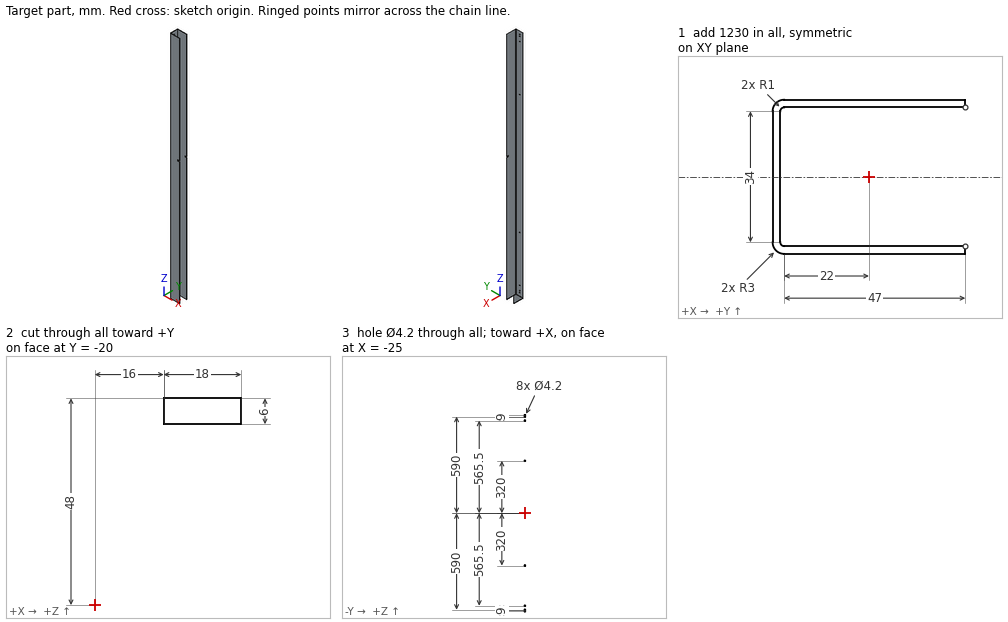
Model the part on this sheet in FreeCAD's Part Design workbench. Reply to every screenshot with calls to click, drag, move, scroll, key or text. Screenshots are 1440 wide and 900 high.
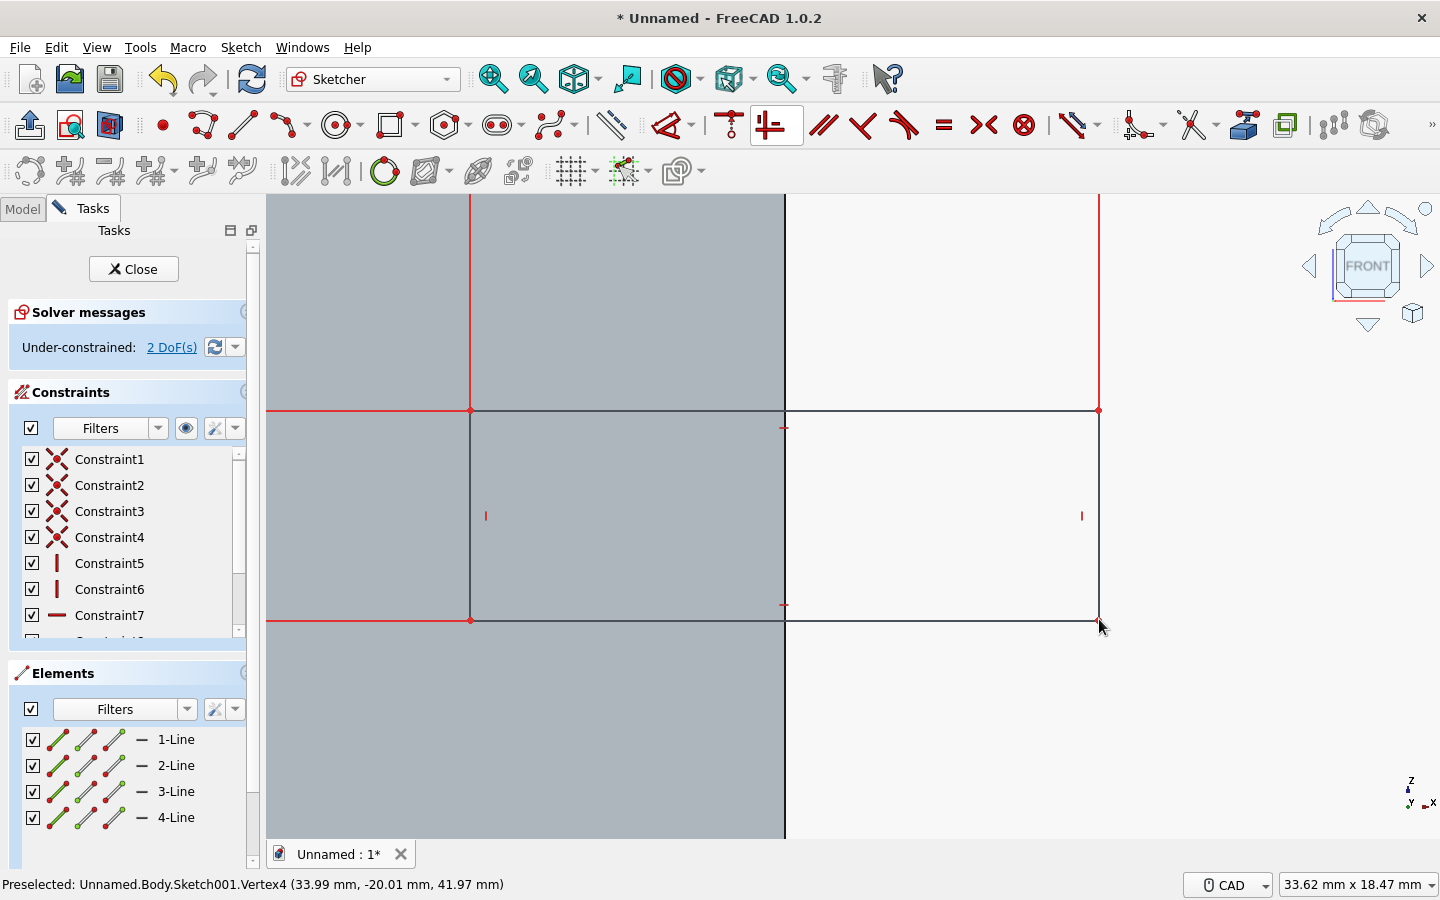
key(d)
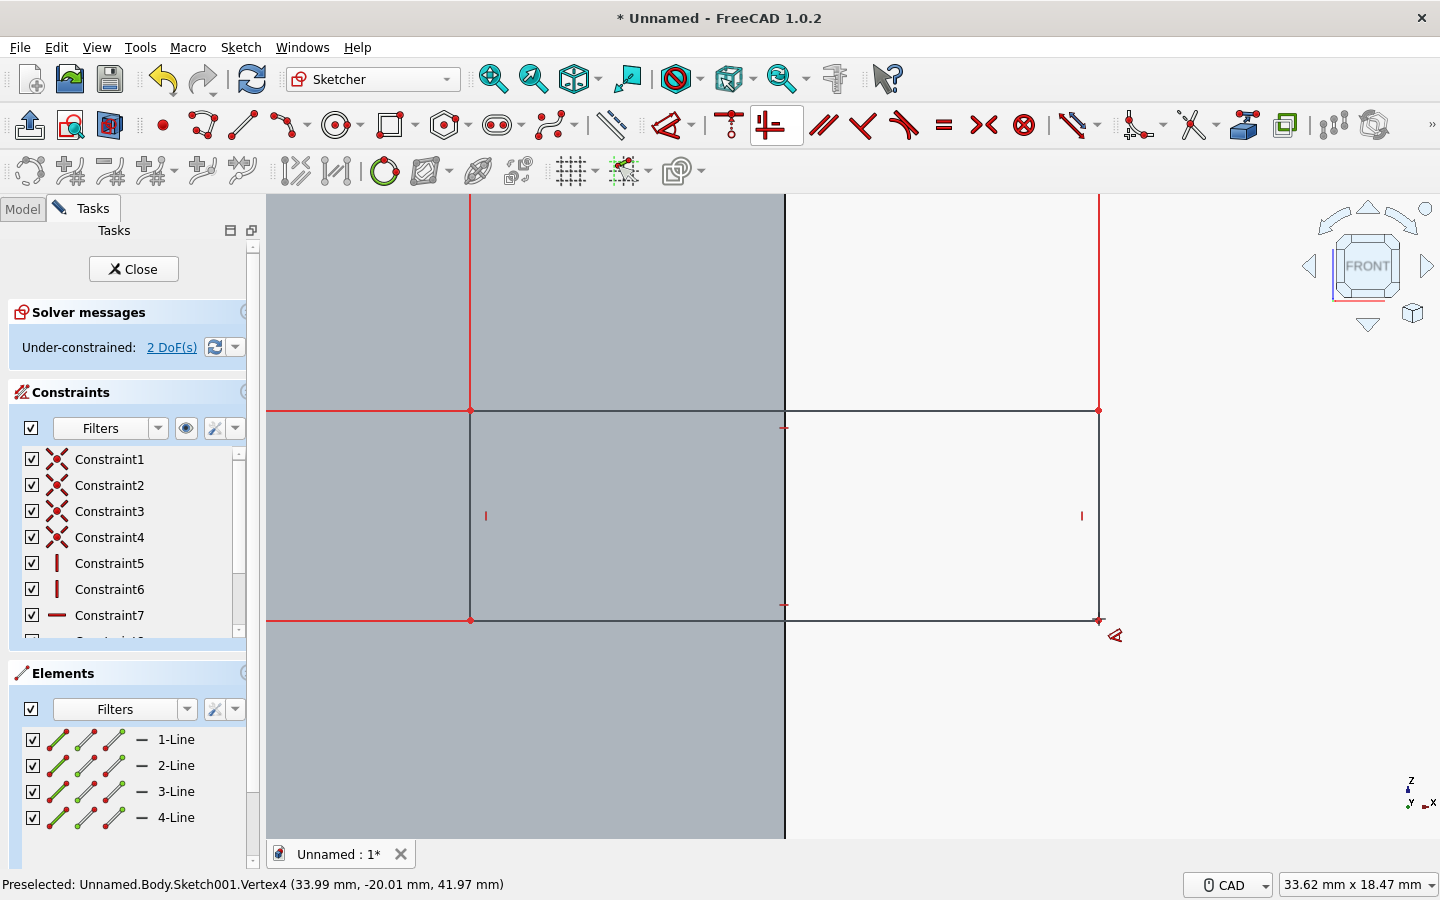
click(470, 411)
click(382, 377)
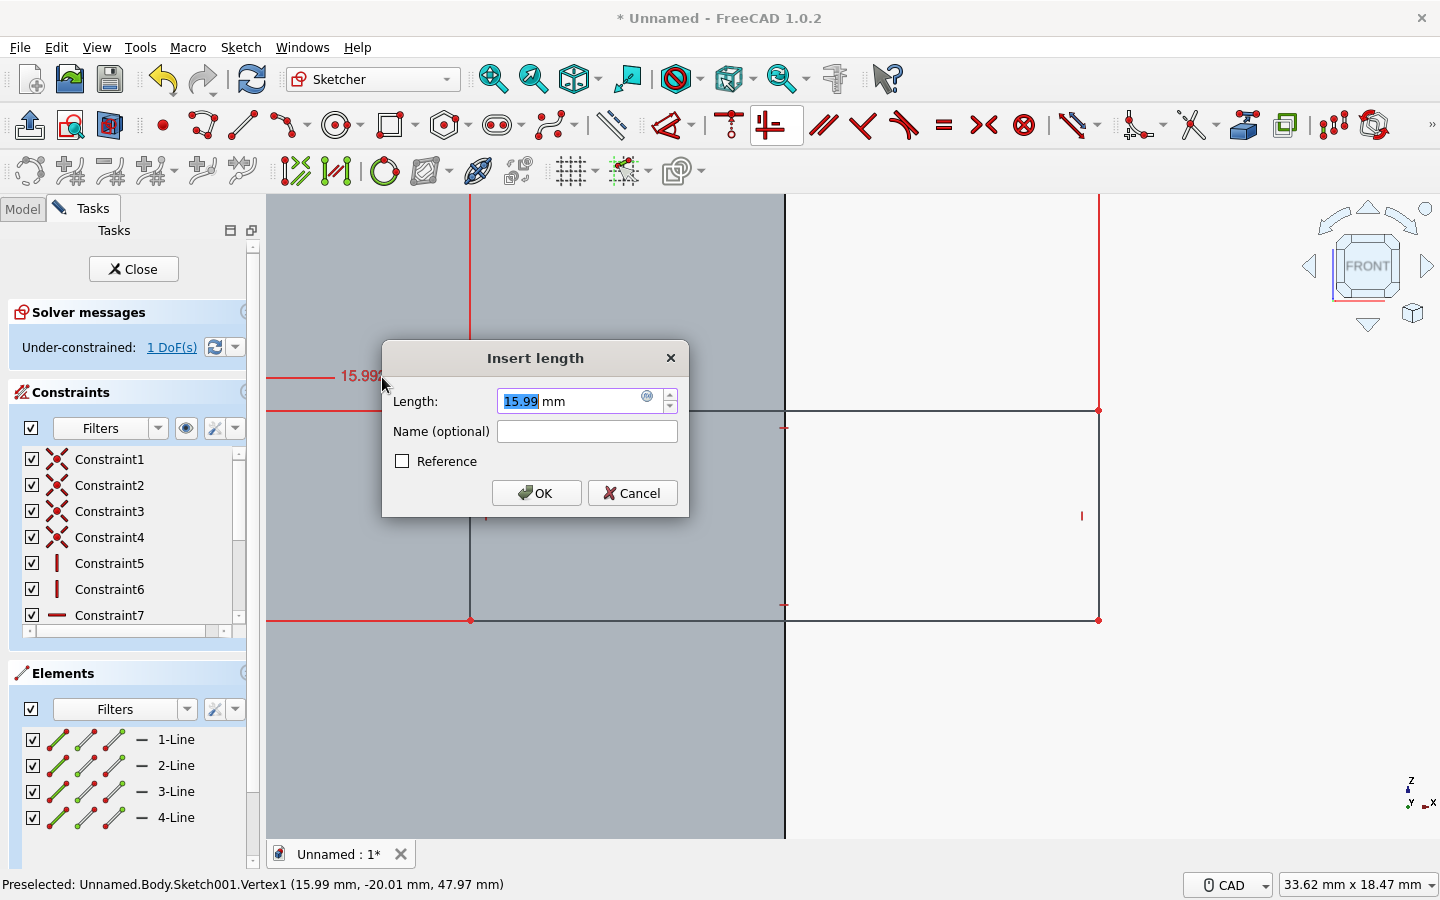
text(16)
key(Return)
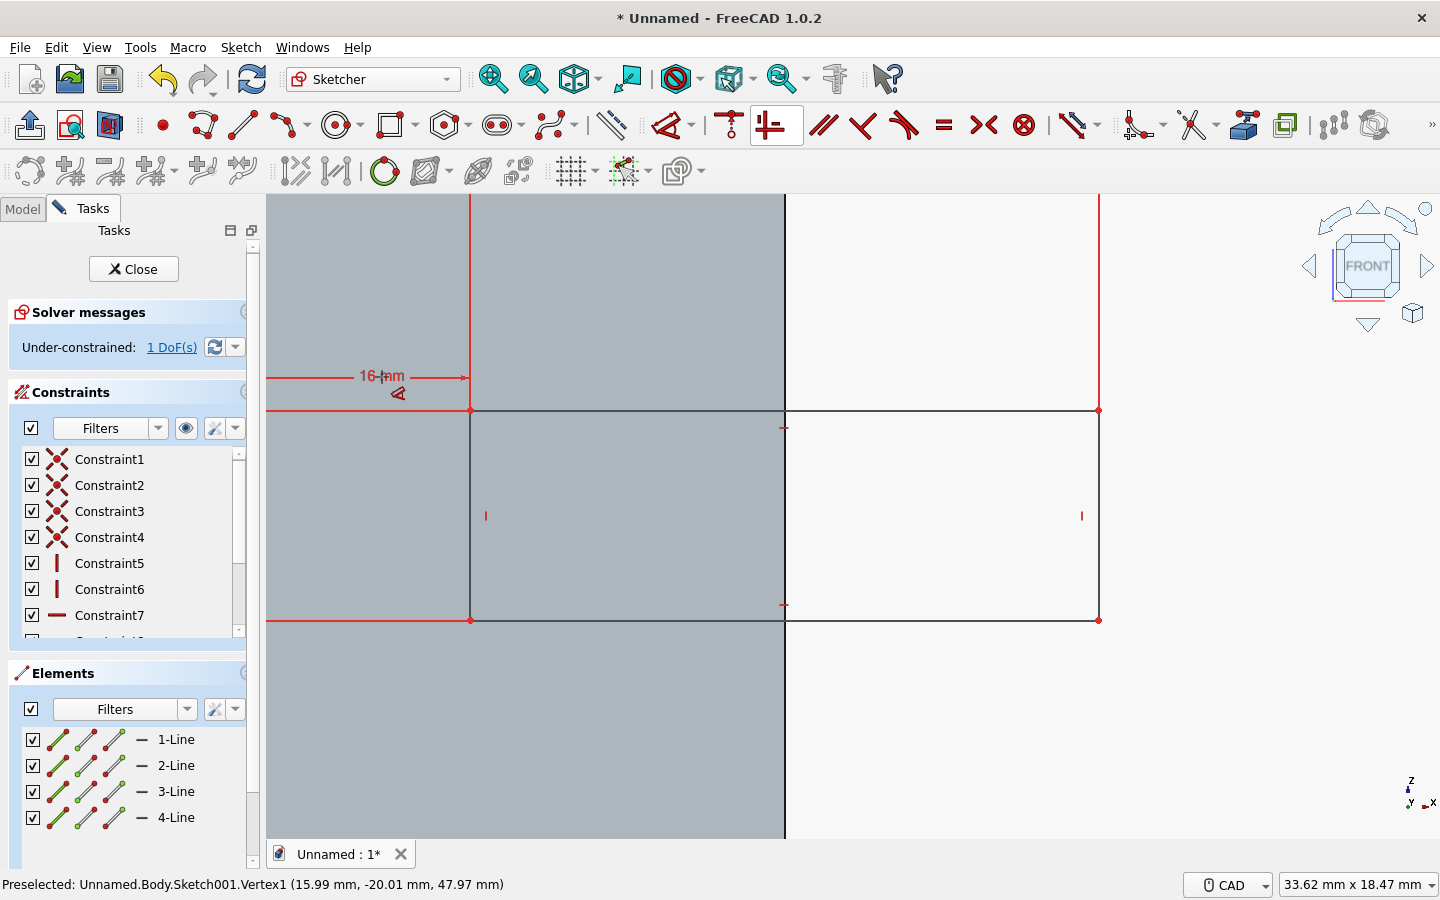
click(470, 411)
click(504, 519)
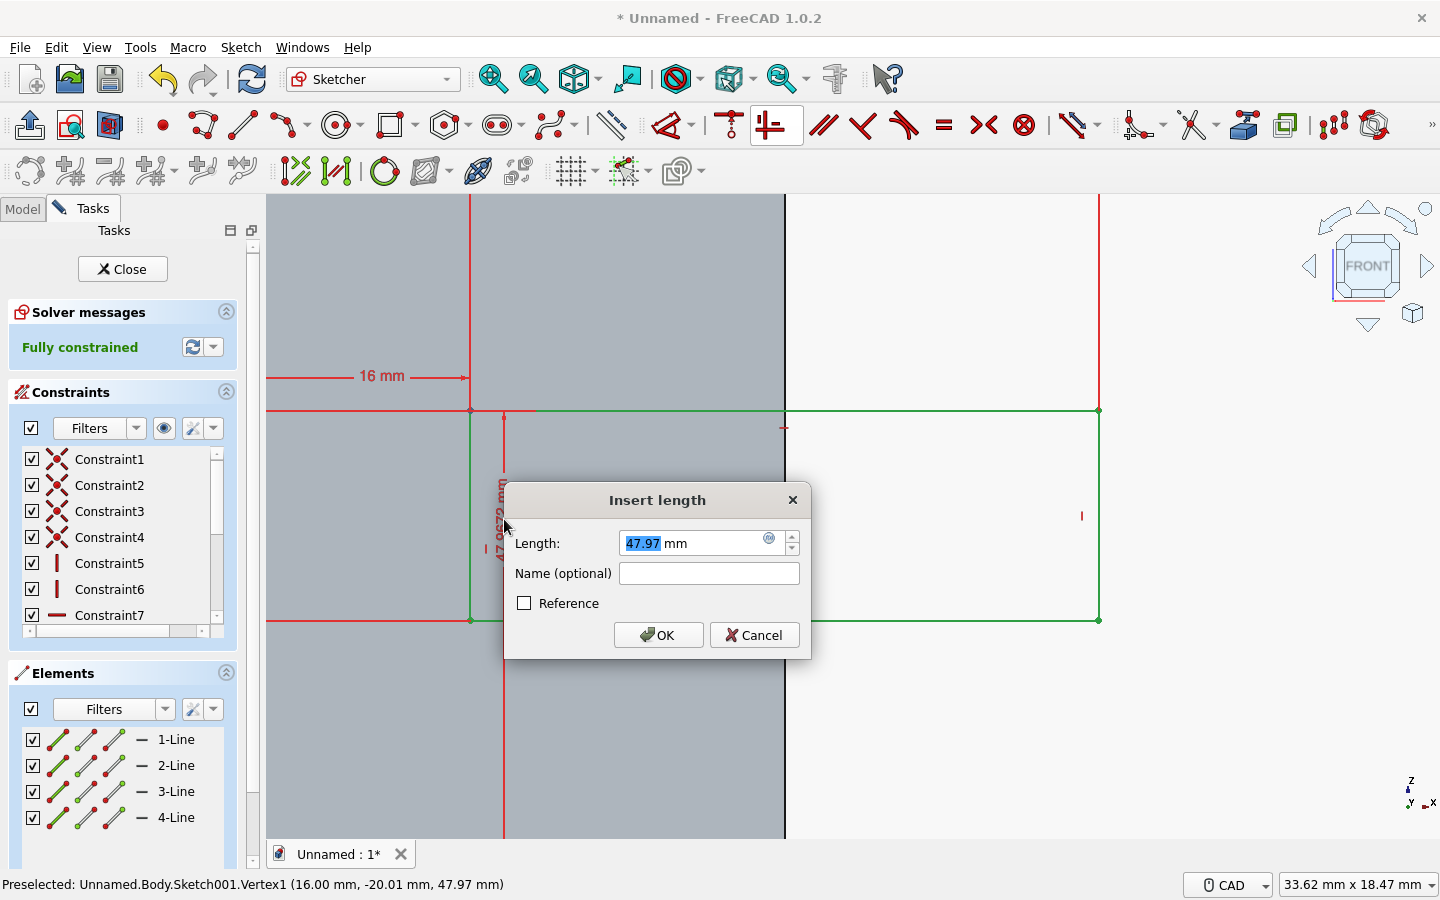
text(48)
key(Return)
key(Escape)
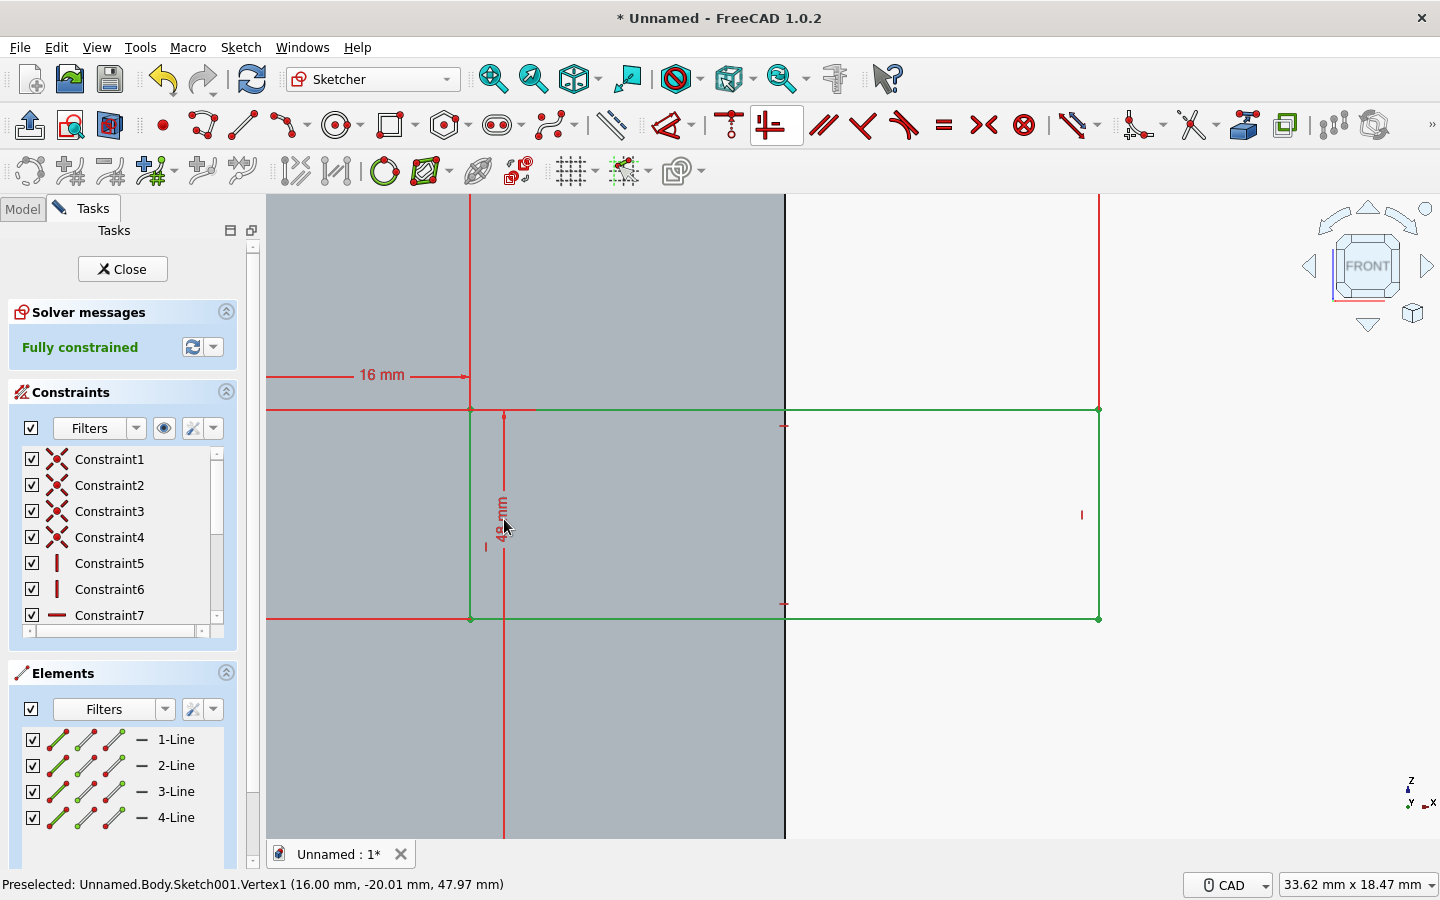
click(123, 269)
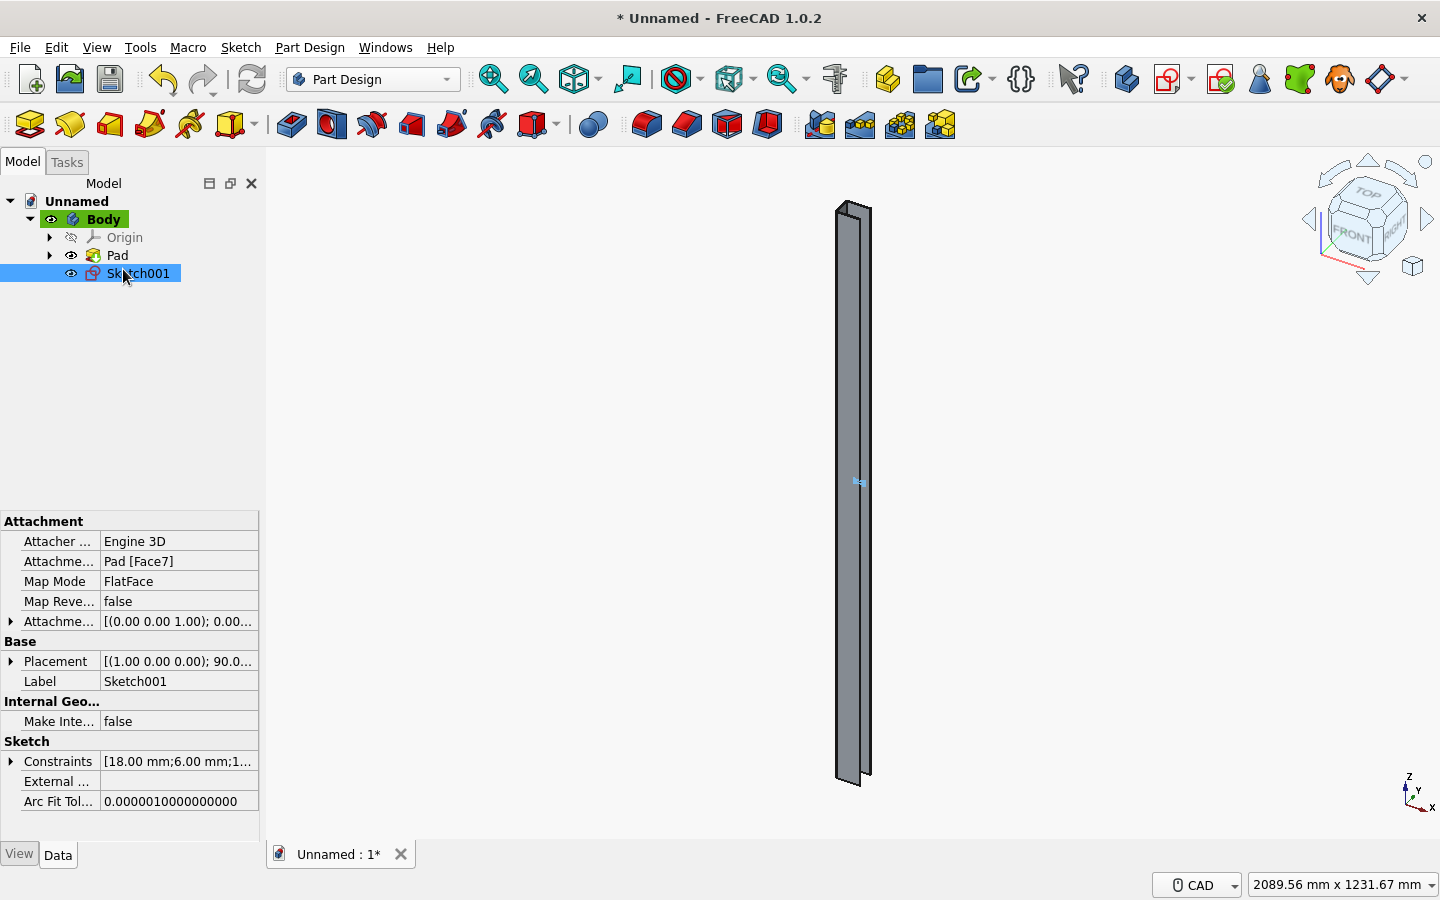
click(292, 124)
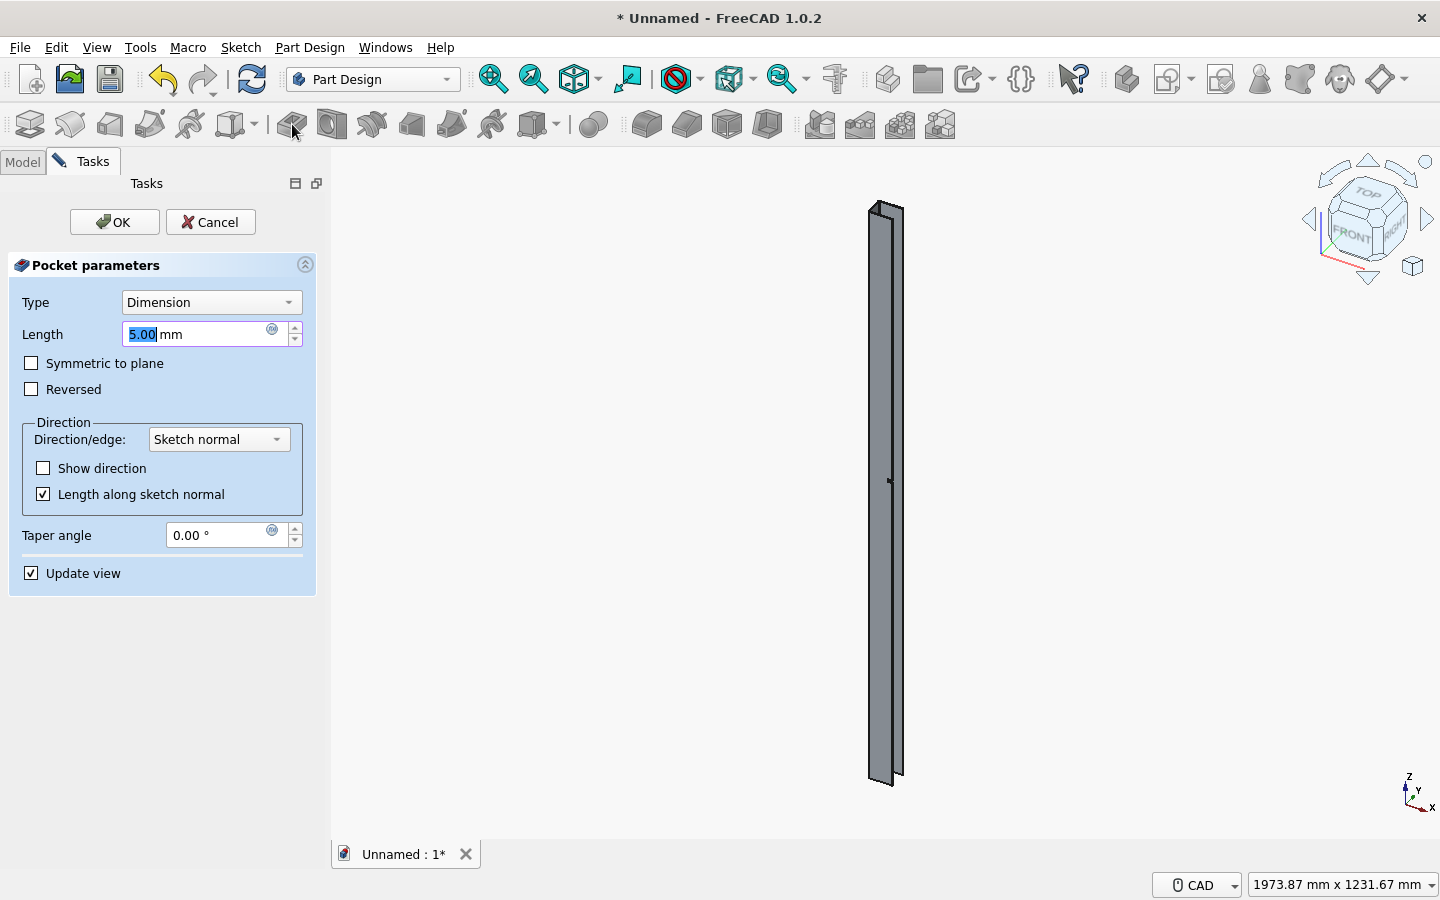
click(212, 302)